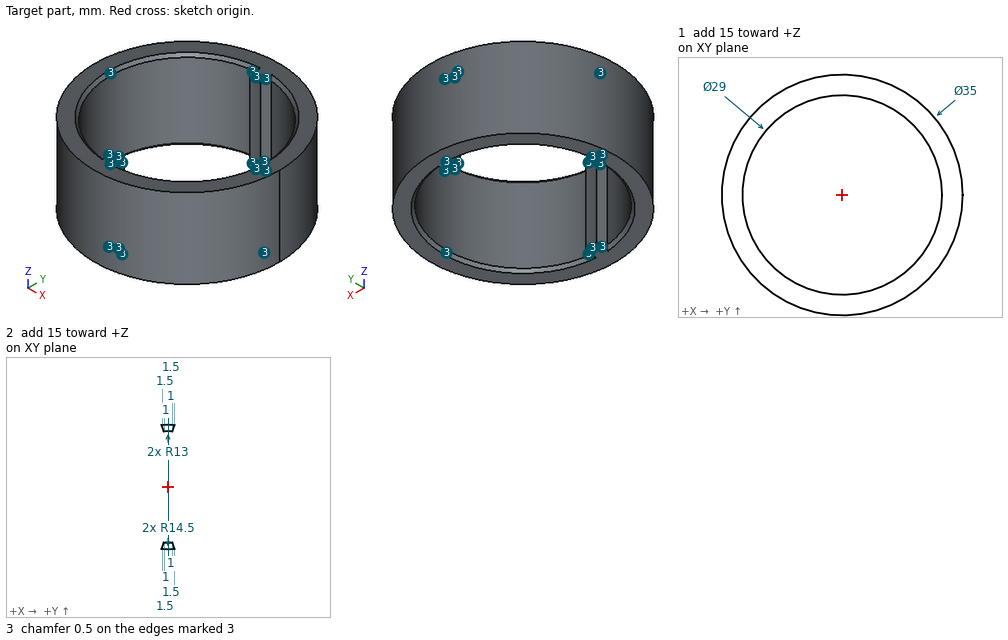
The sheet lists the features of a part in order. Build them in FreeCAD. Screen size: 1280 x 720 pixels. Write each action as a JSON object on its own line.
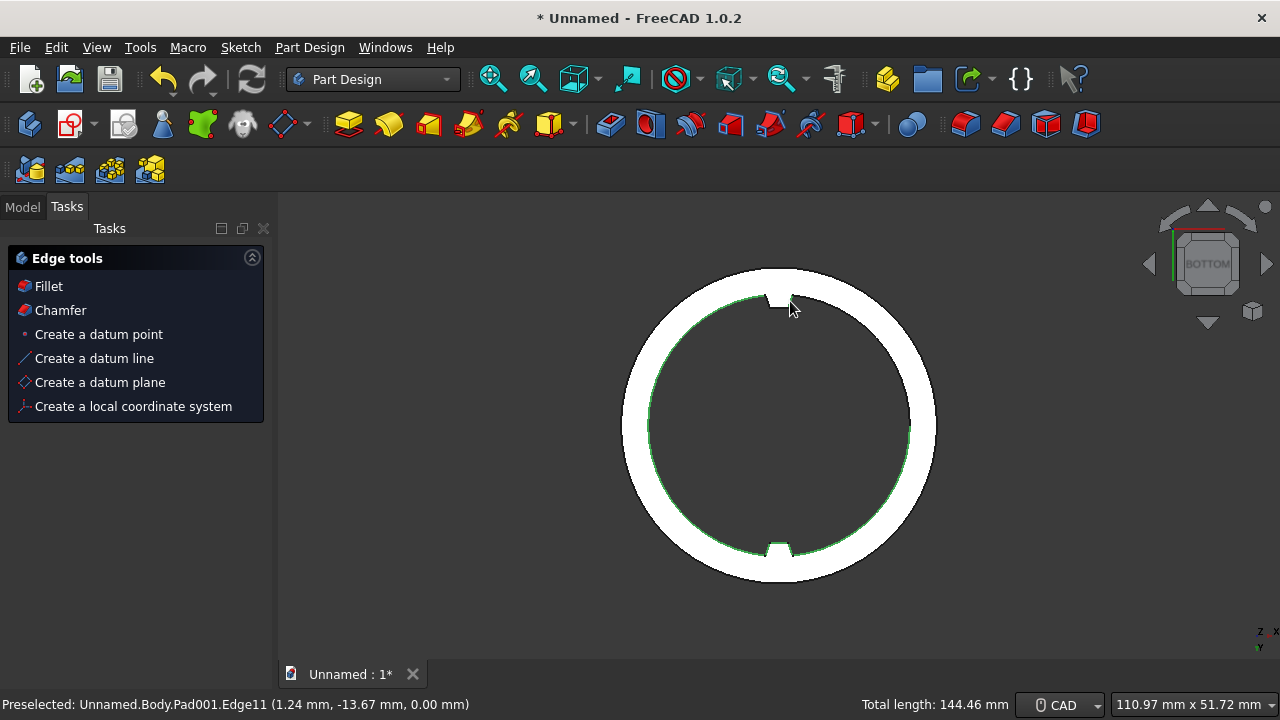
{"action": "left_click", "coordinate": [768, 301], "text": "ctrl"}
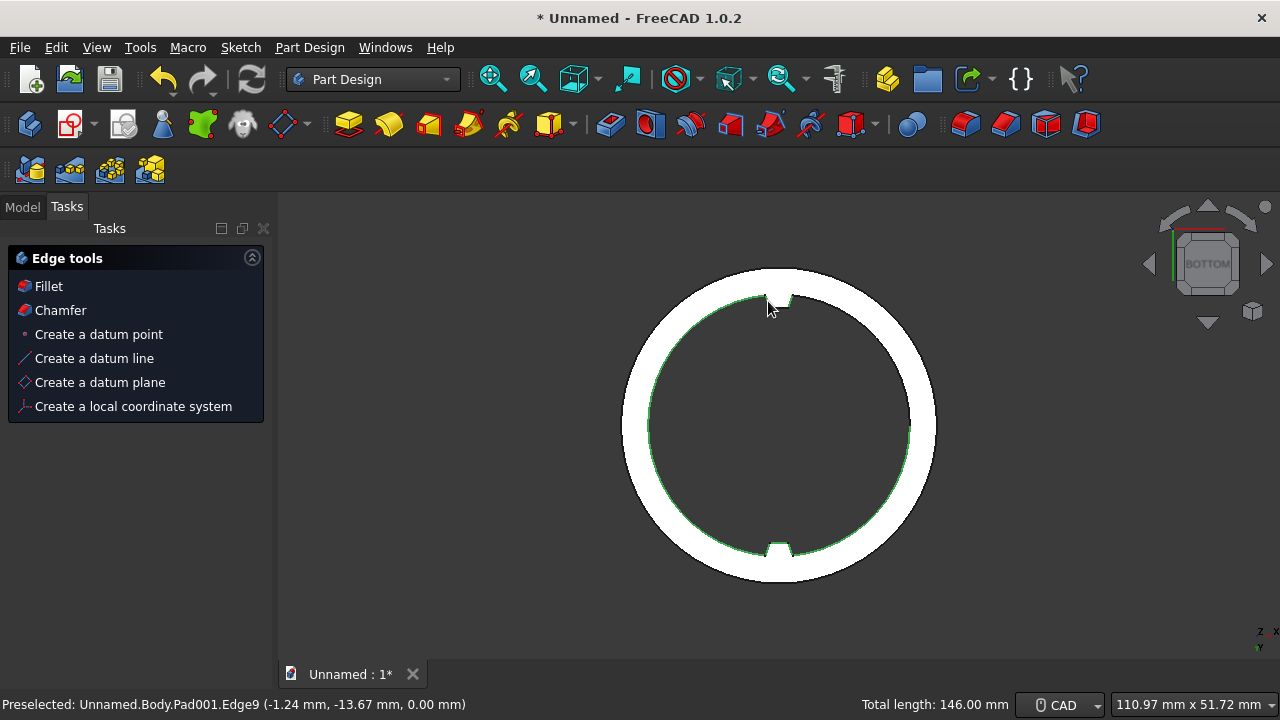
{"action": "scroll", "coordinate": [779, 307], "scroll_direction": "up", "scroll_amount": 4}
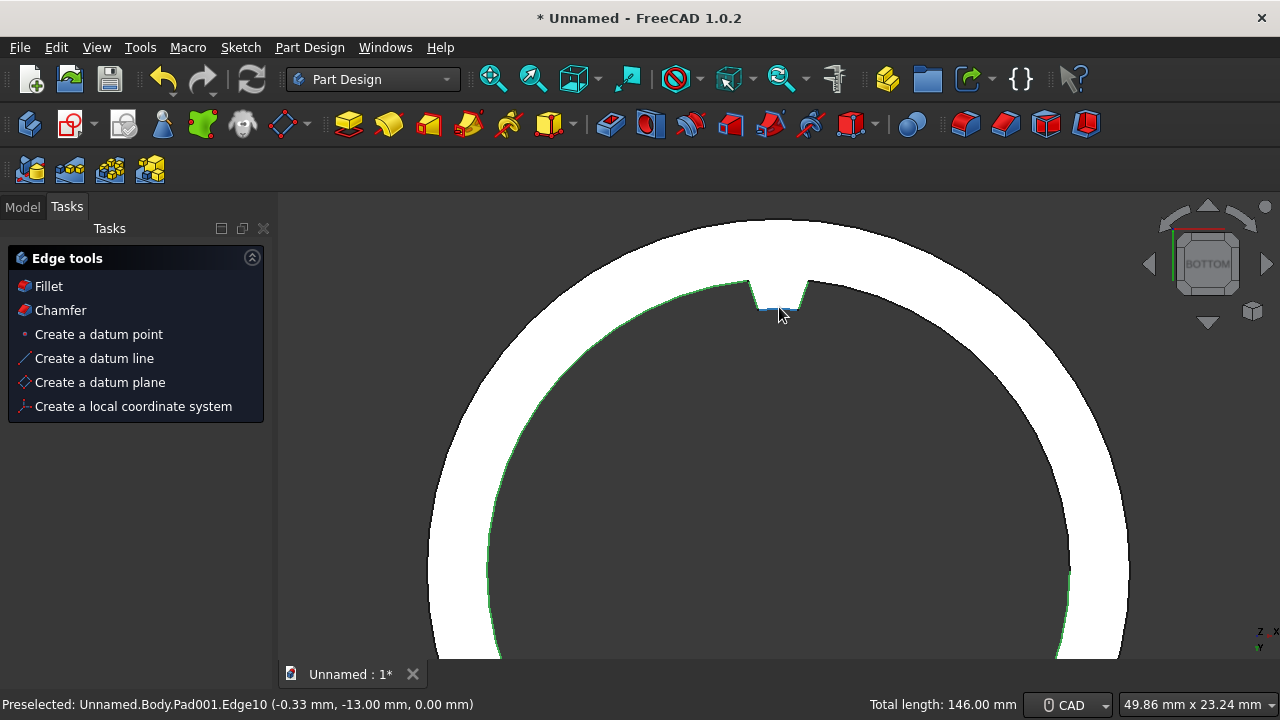
{"action": "left_click", "coordinate": [770, 308], "text": "ctrl"}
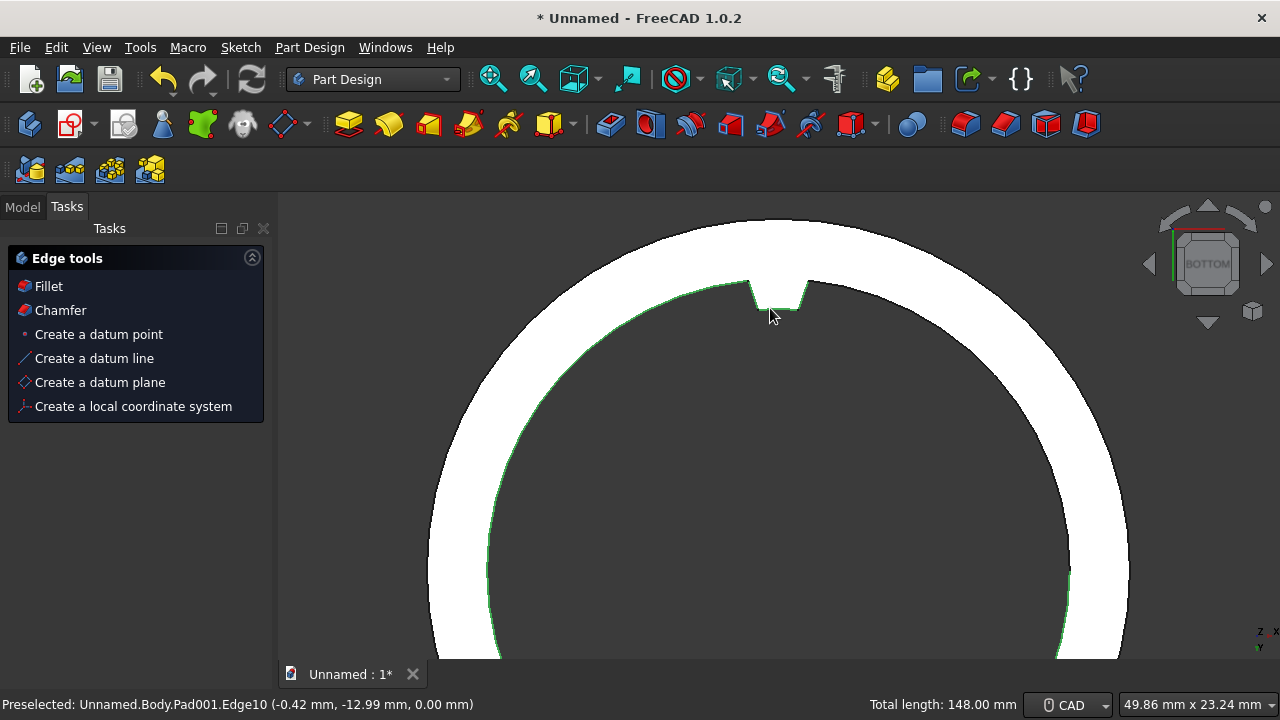
{"action": "left_click", "coordinate": [1006, 124]}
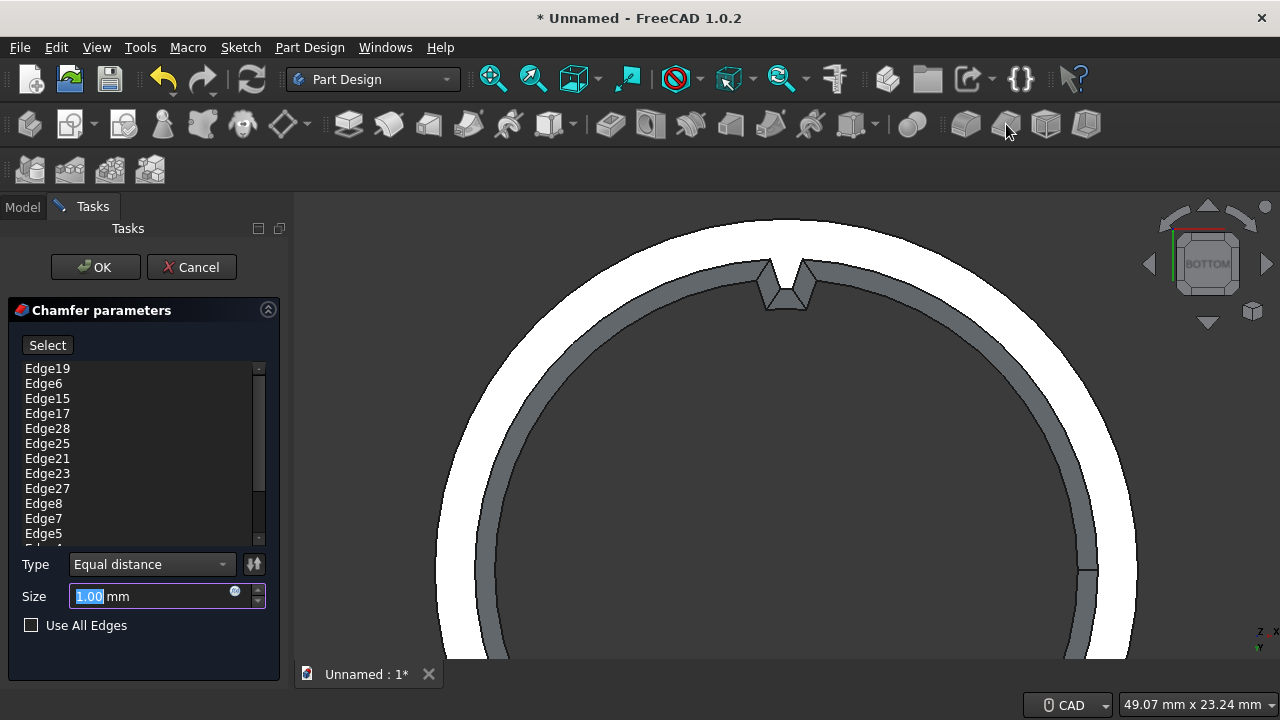
{"action": "type", "text": "0.5"}
{"action": "key", "text": "Tab"}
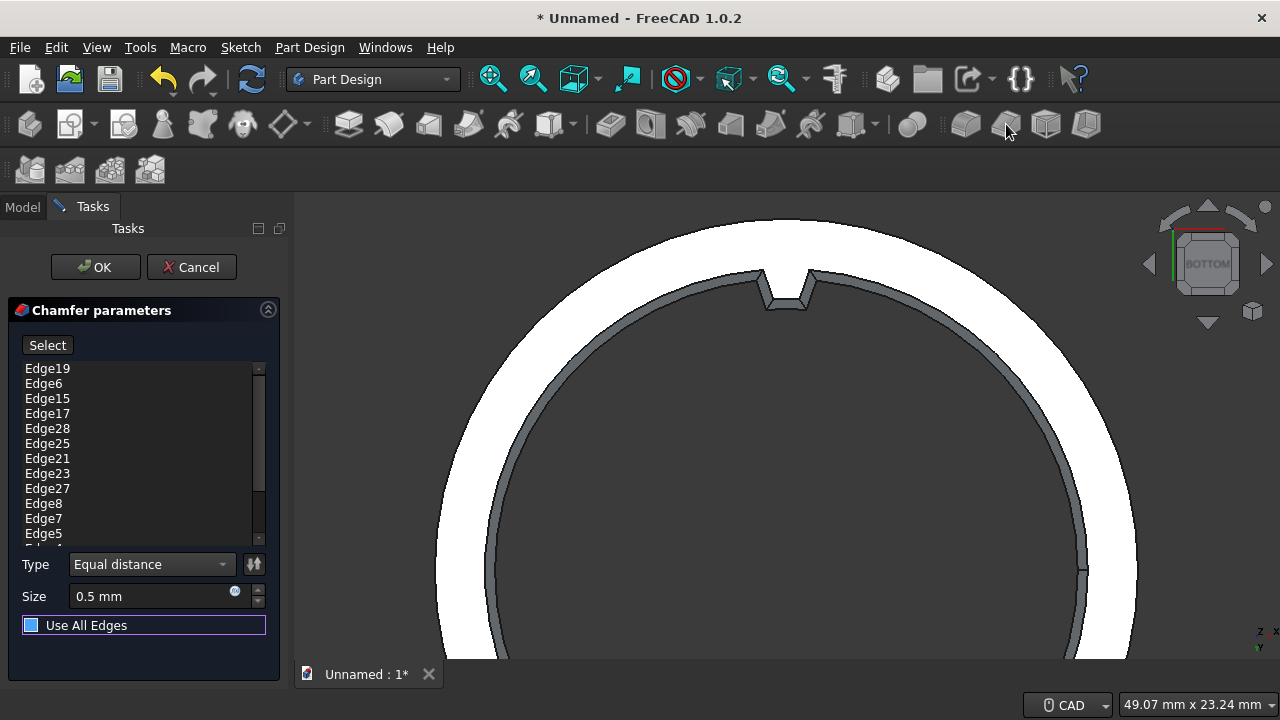
{"action": "left_click", "coordinate": [96, 267]}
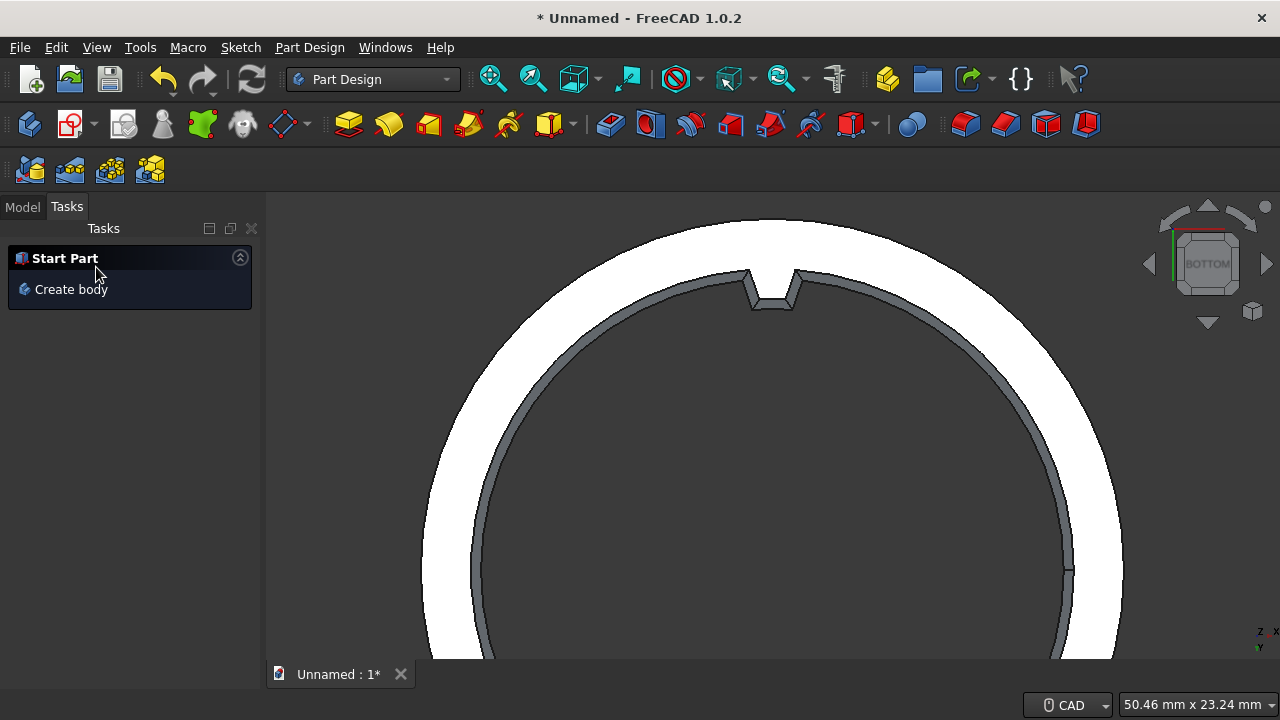
{"action": "key", "text": "0"}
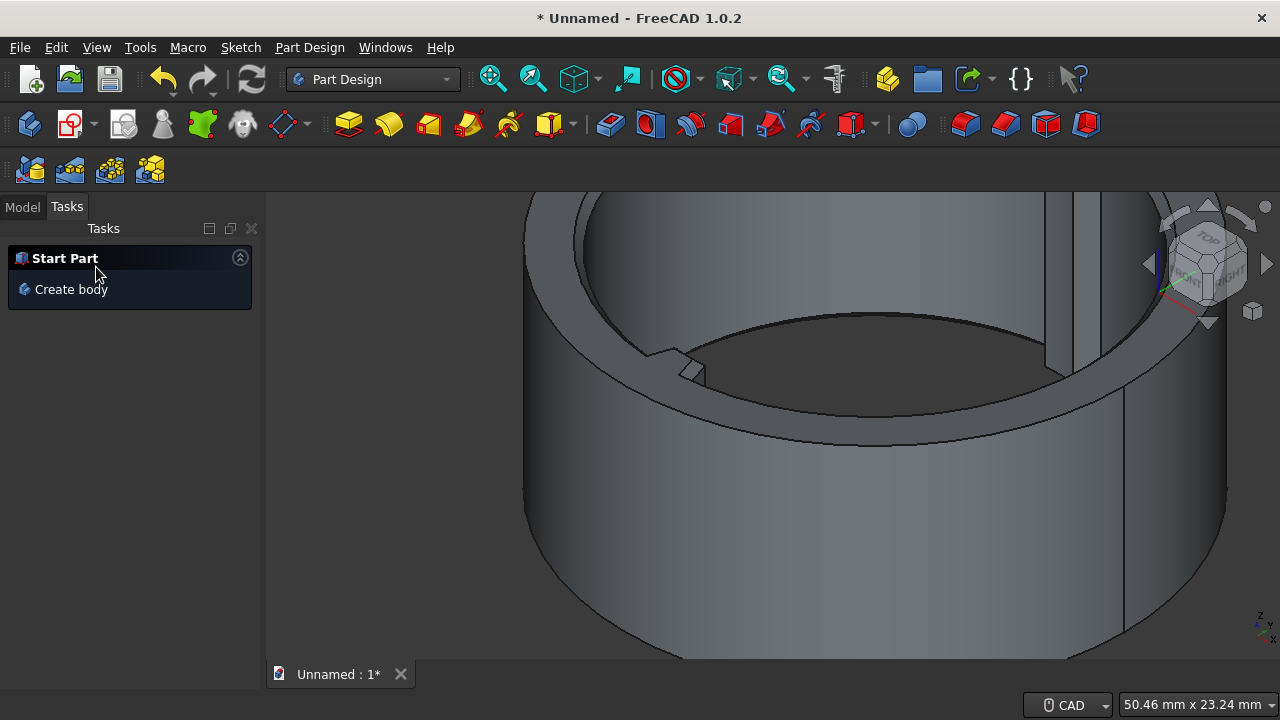
{"action": "left_click", "coordinate": [494, 80]}